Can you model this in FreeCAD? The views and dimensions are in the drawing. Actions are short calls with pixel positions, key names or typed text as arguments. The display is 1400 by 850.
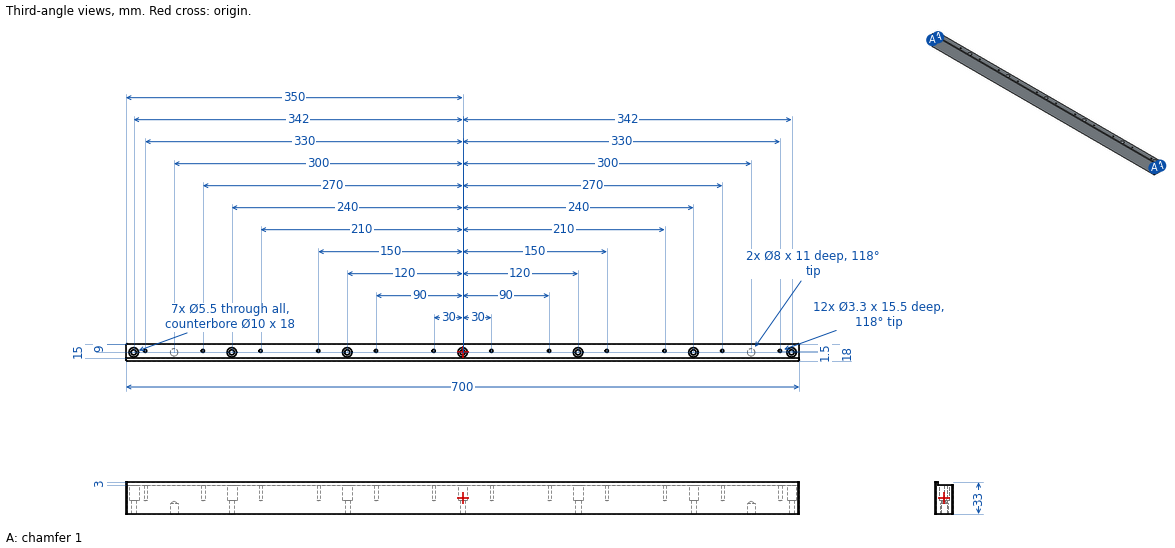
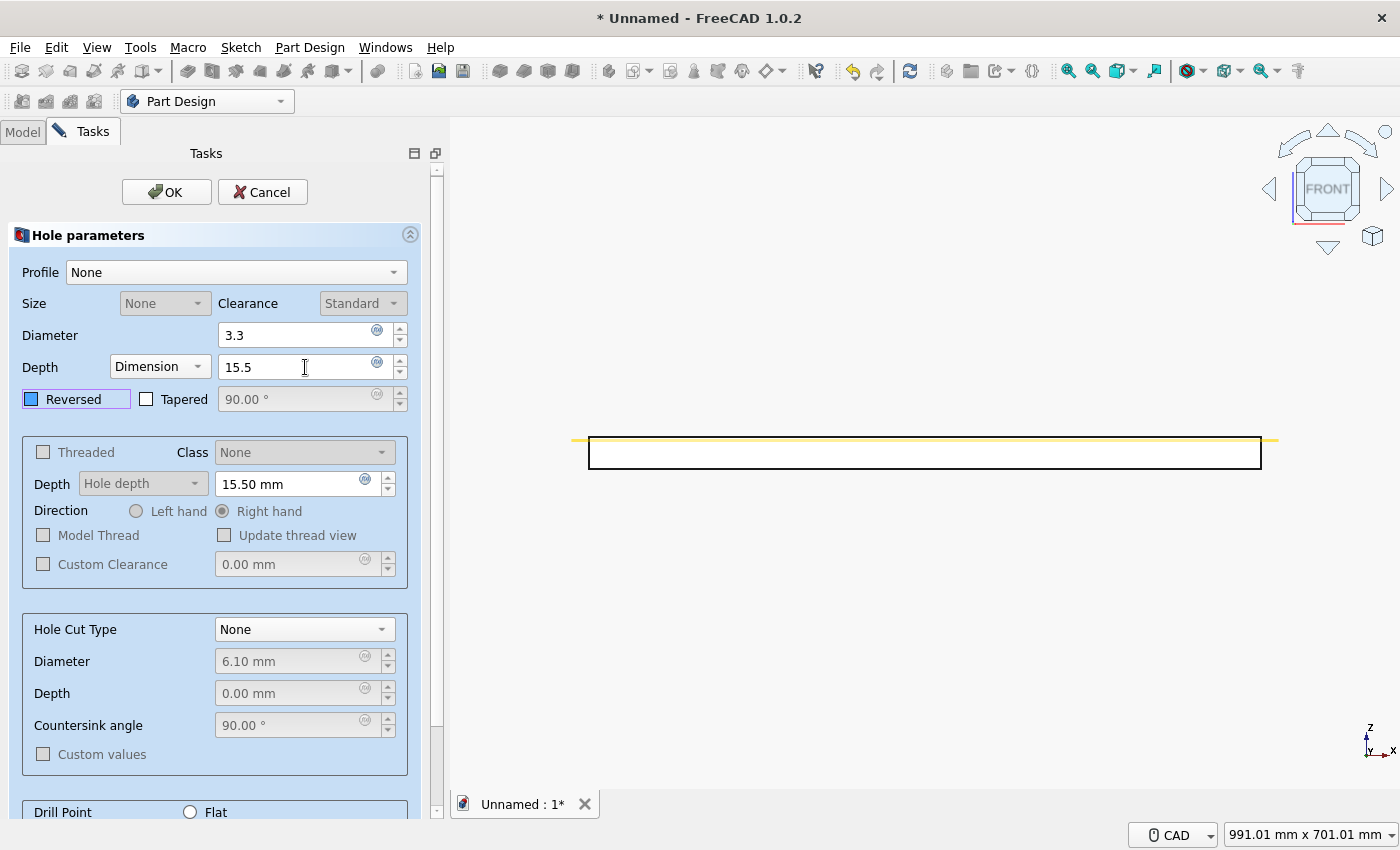
click(167, 192)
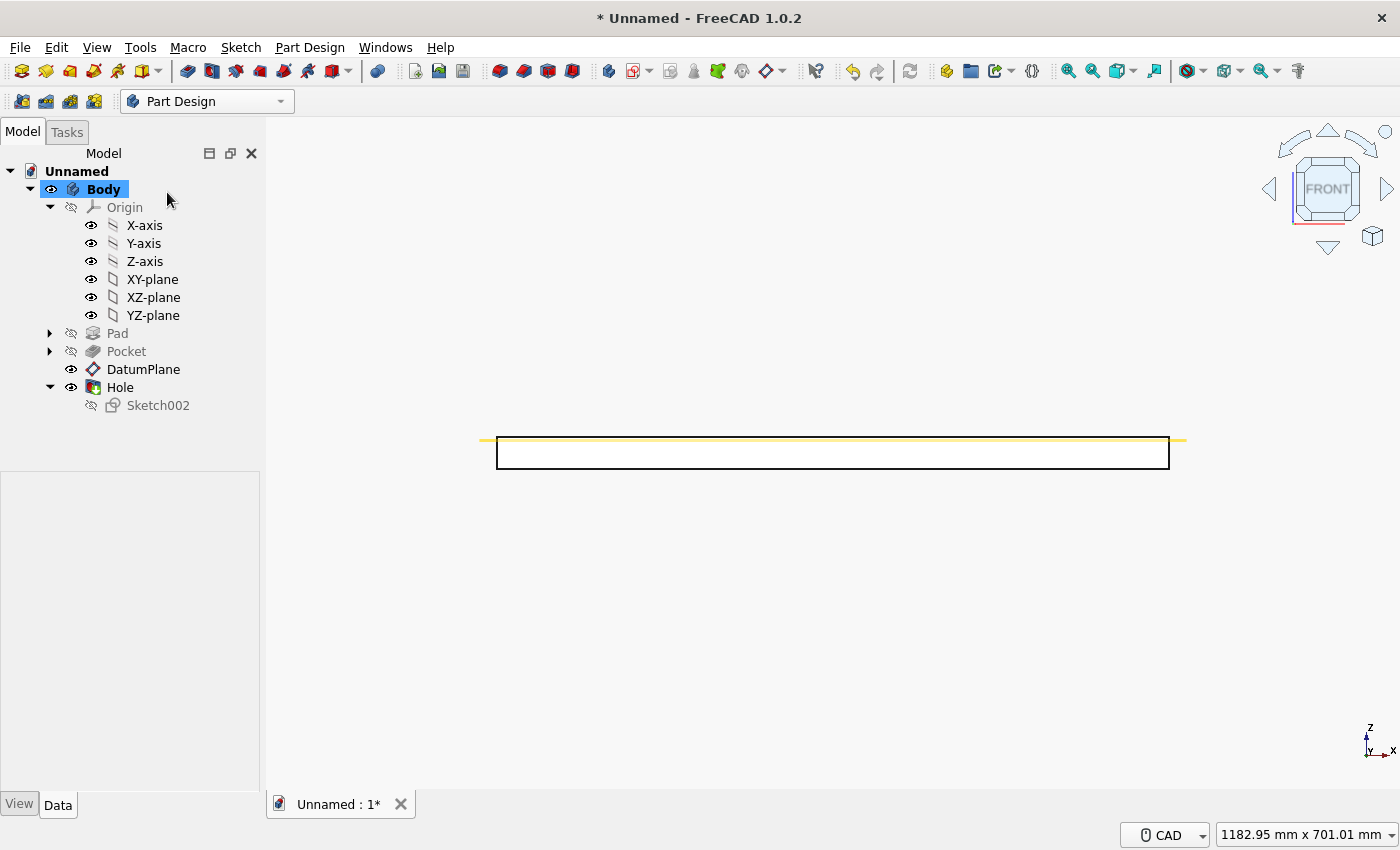
click(116, 369)
key(space)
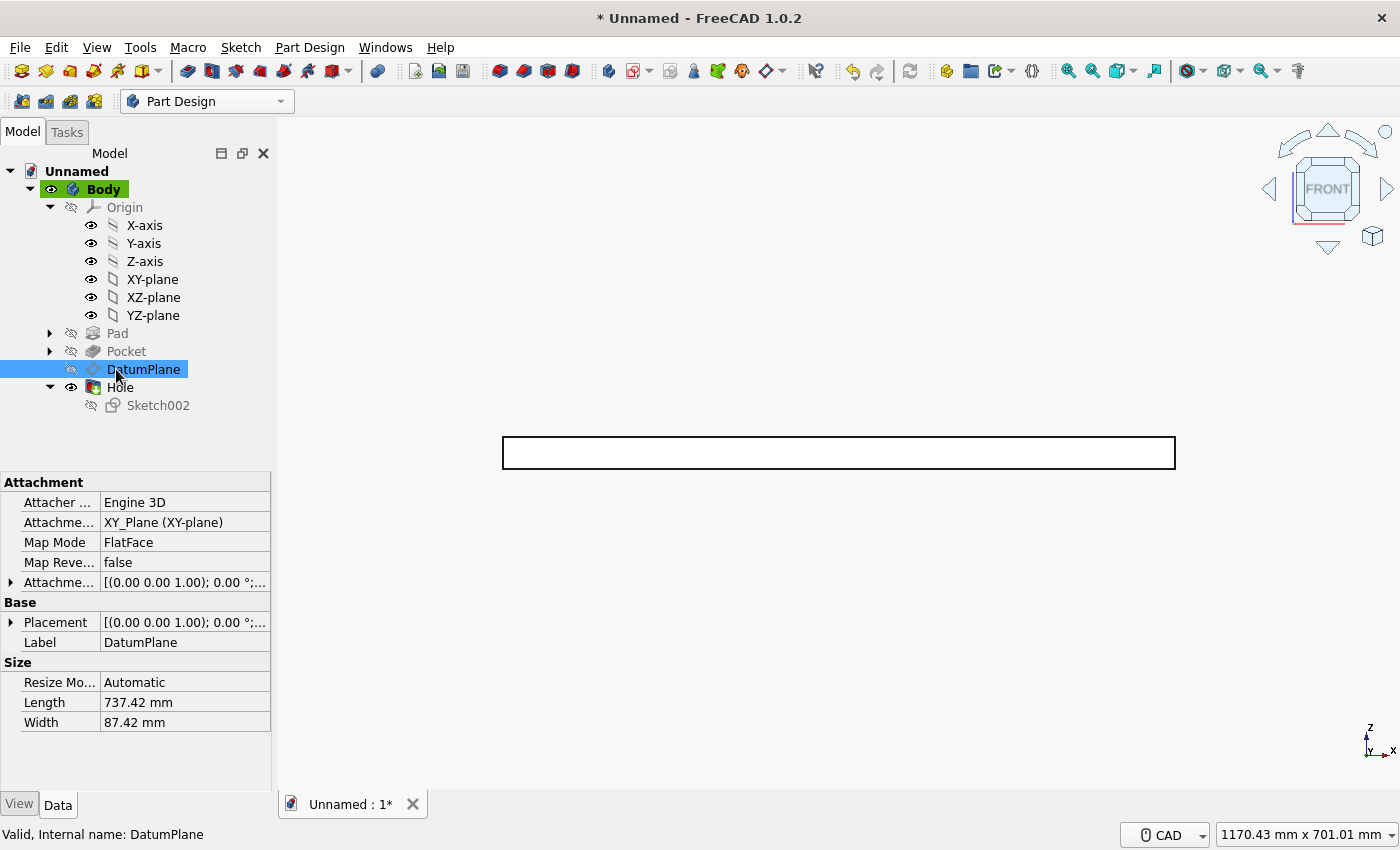
key(0)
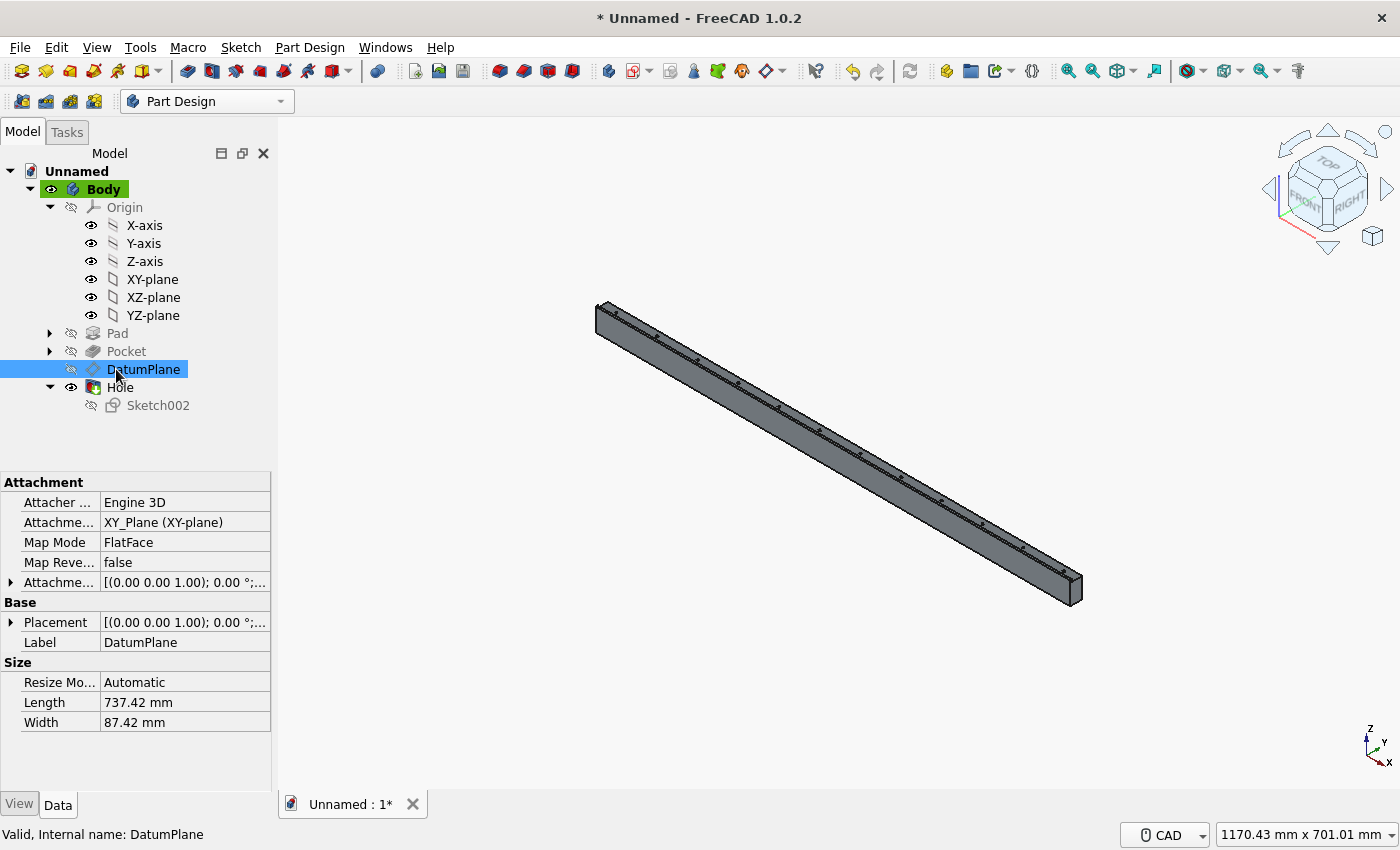
scroll(1037, 559, up, 11)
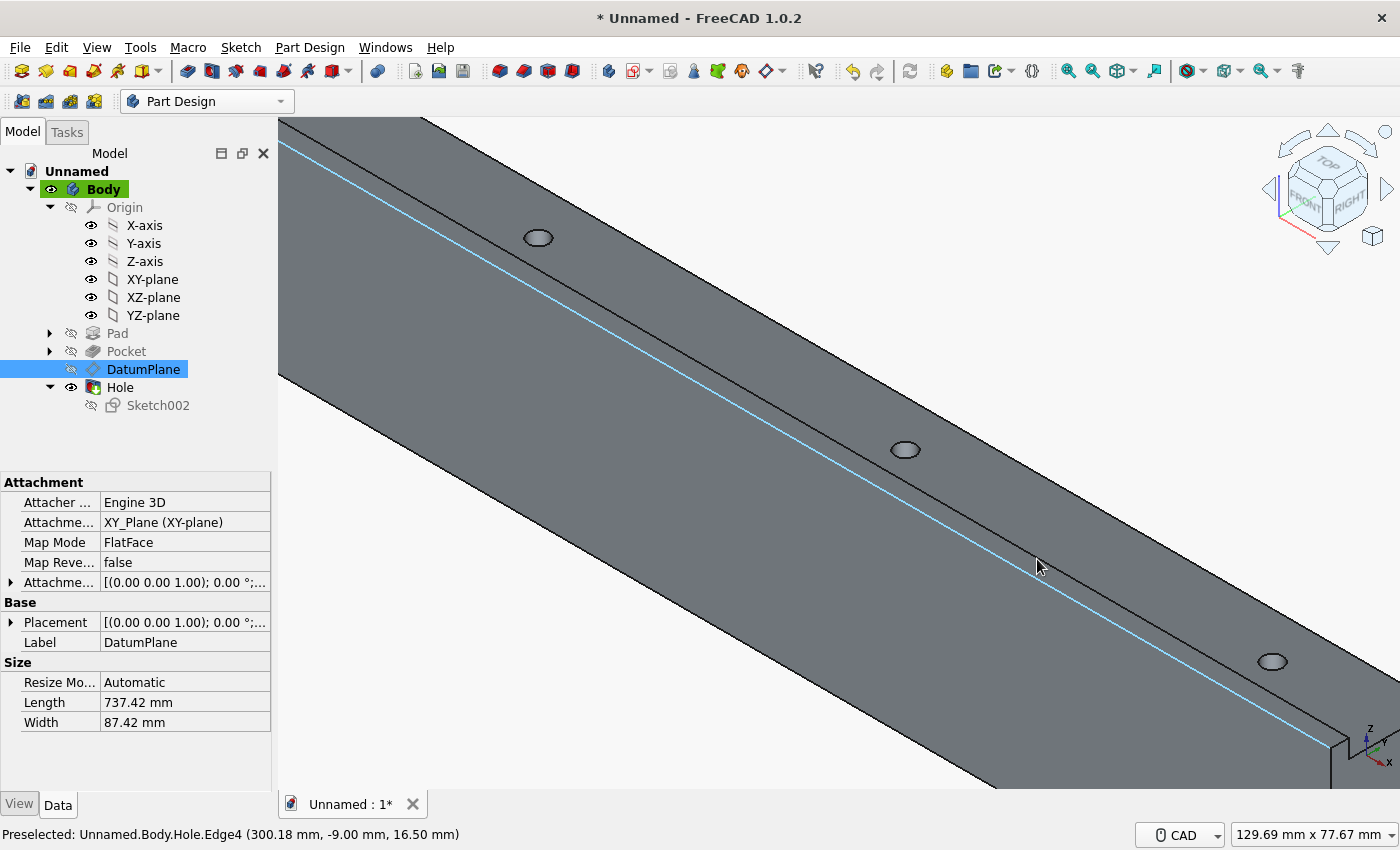
click(422, 212)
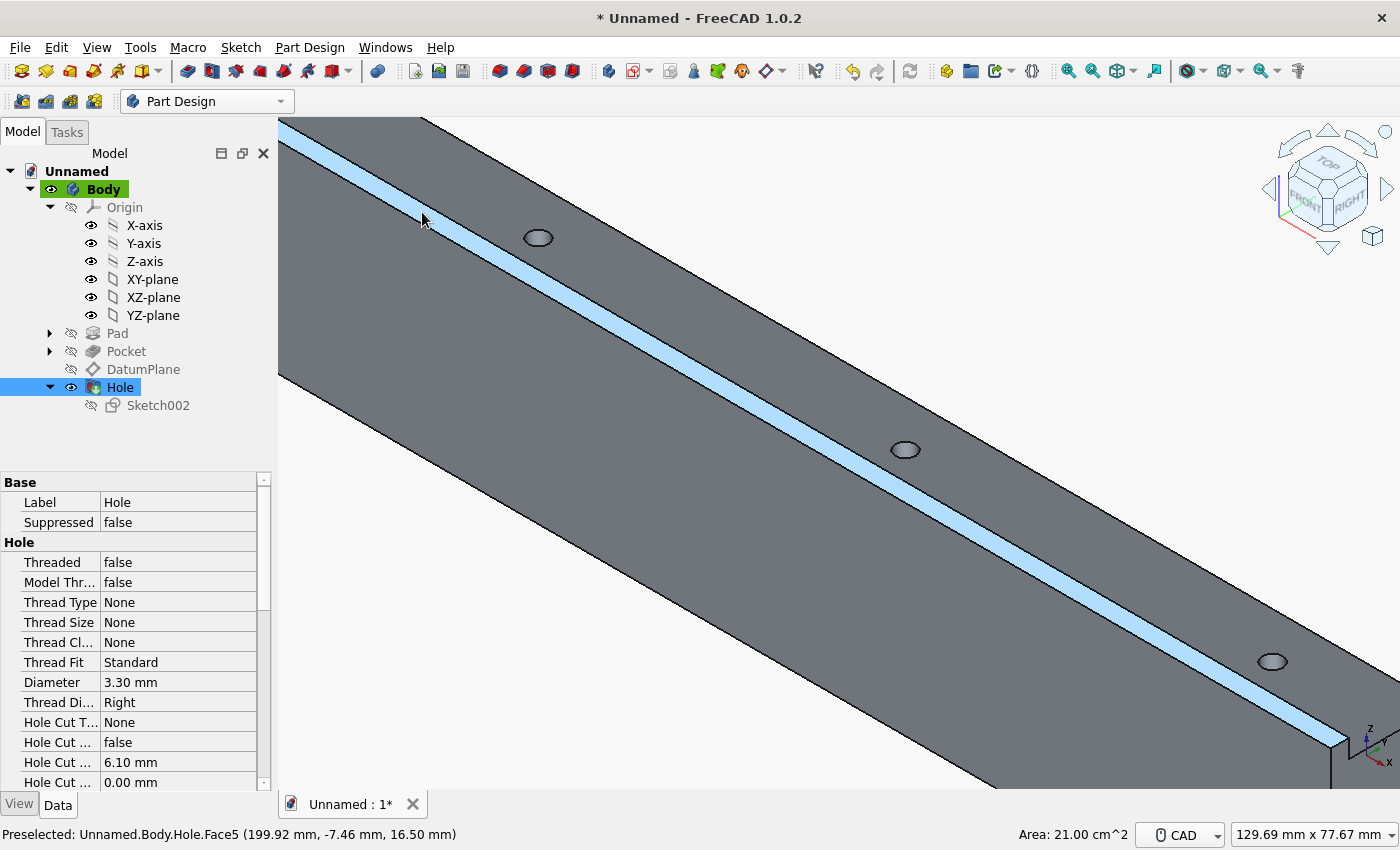
click(634, 72)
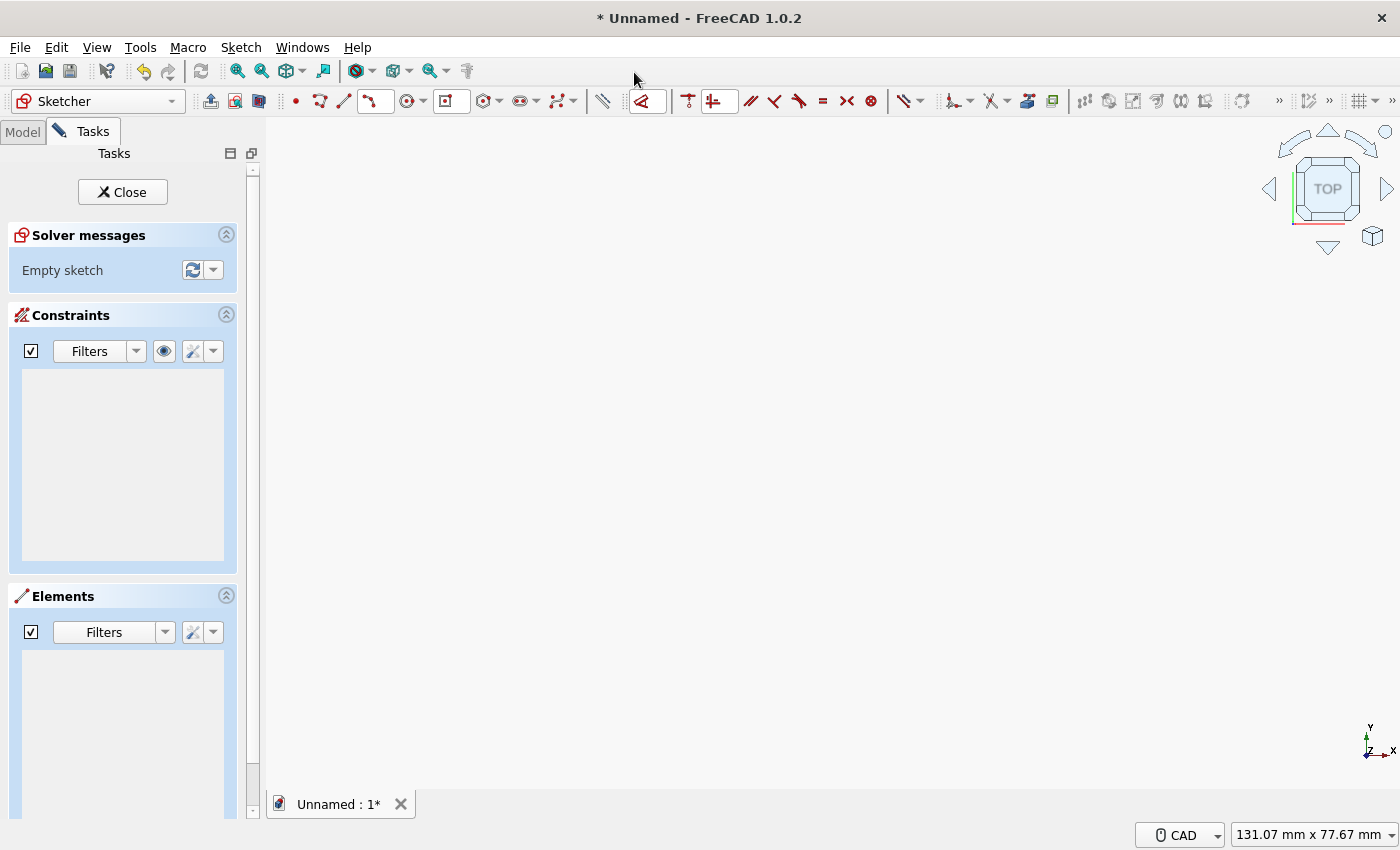
scroll(940, 356, down, 11)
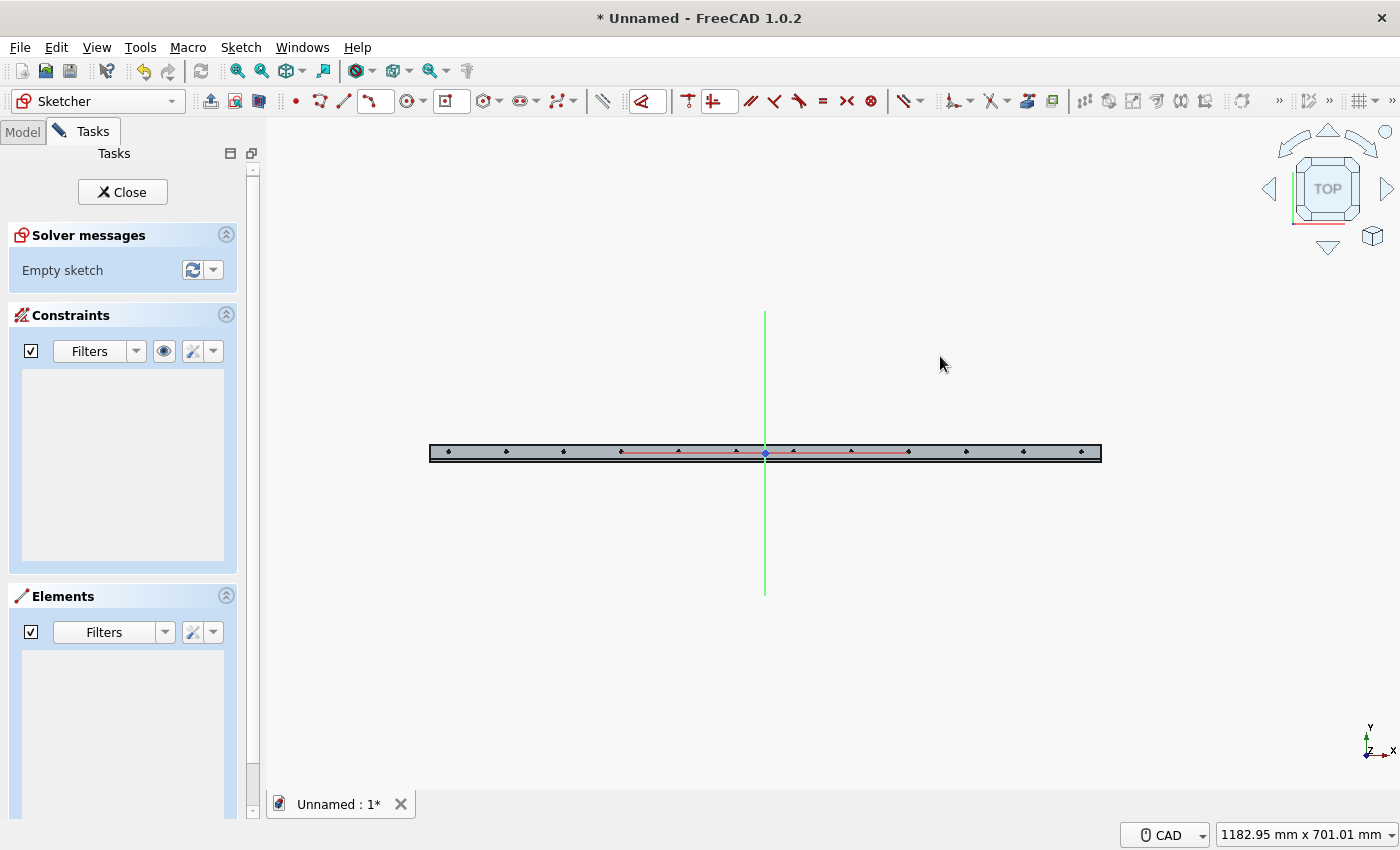
key(g)
key(c)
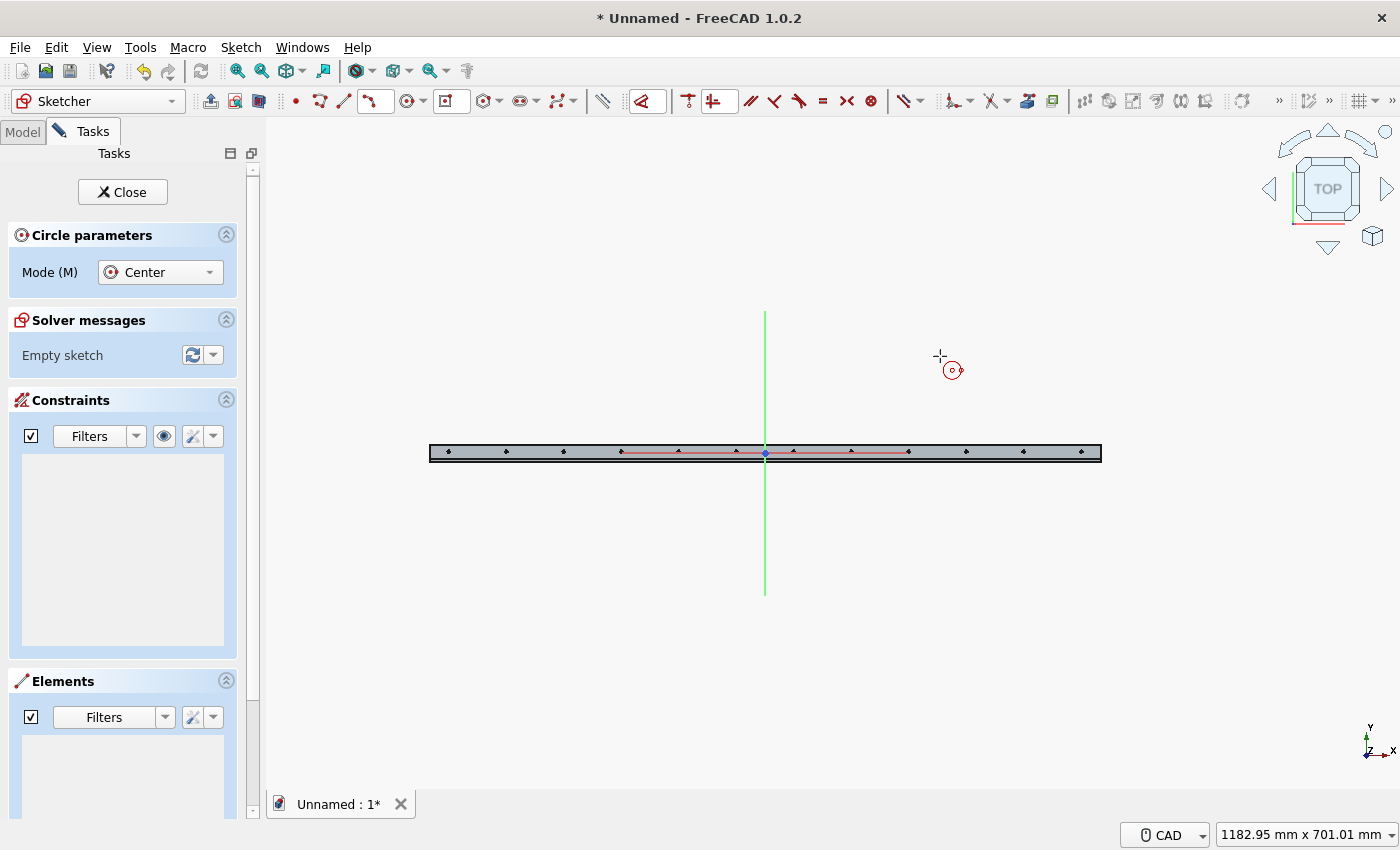
scroll(437, 453, up, 11)